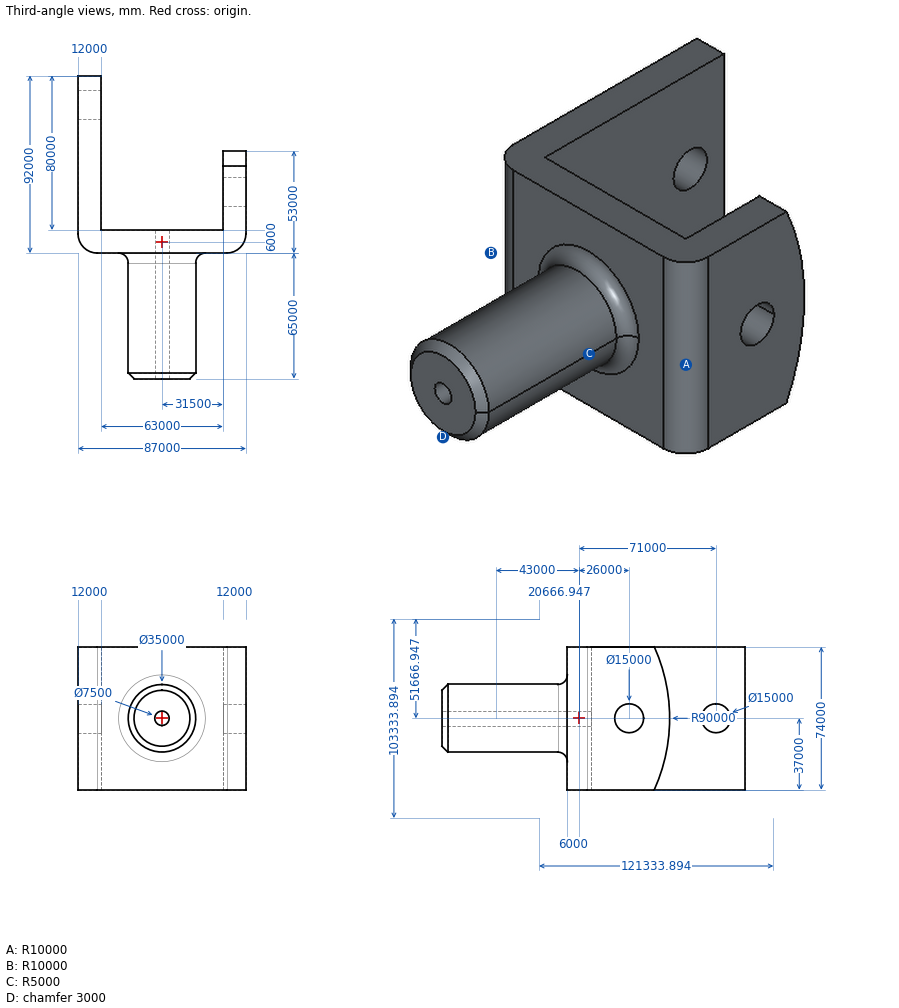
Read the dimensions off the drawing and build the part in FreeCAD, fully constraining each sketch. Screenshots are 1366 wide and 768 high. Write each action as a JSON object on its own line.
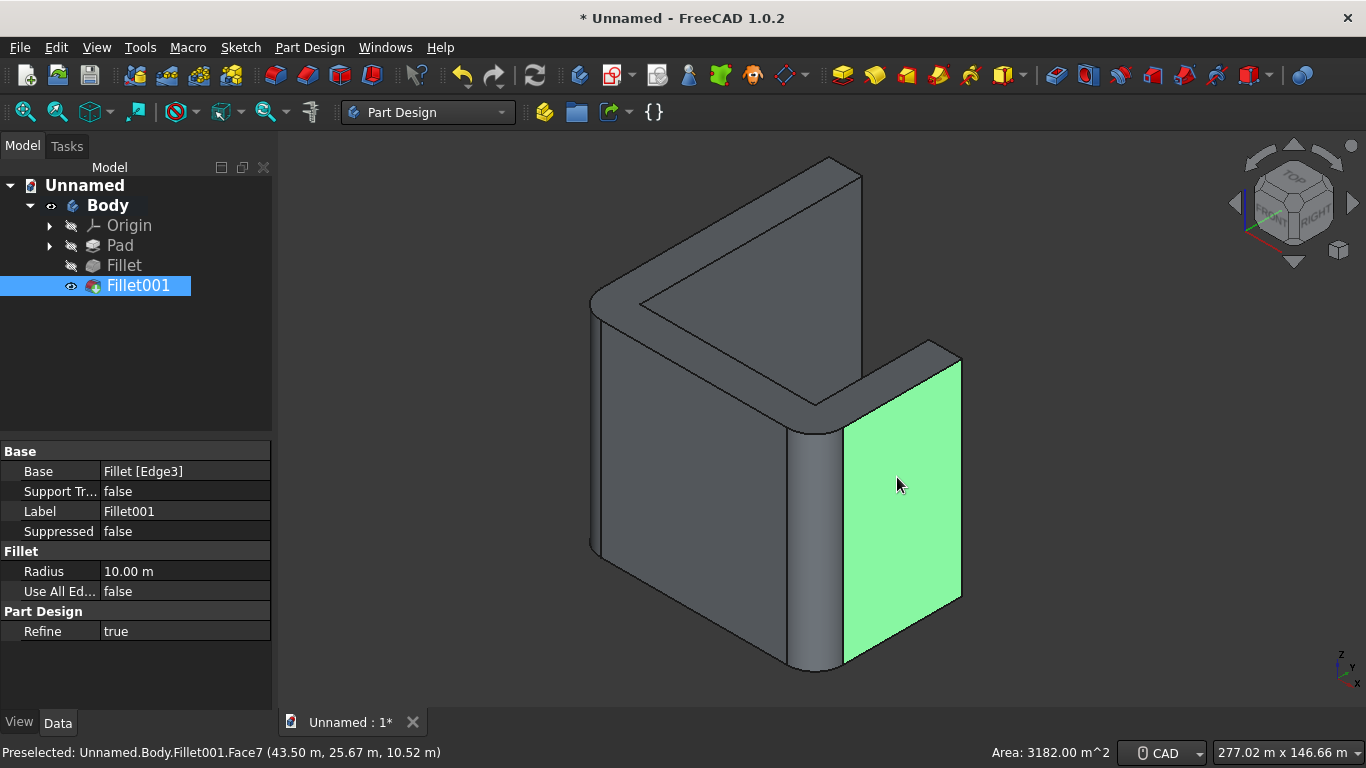
{"action": "left_click", "coordinate": [612, 76]}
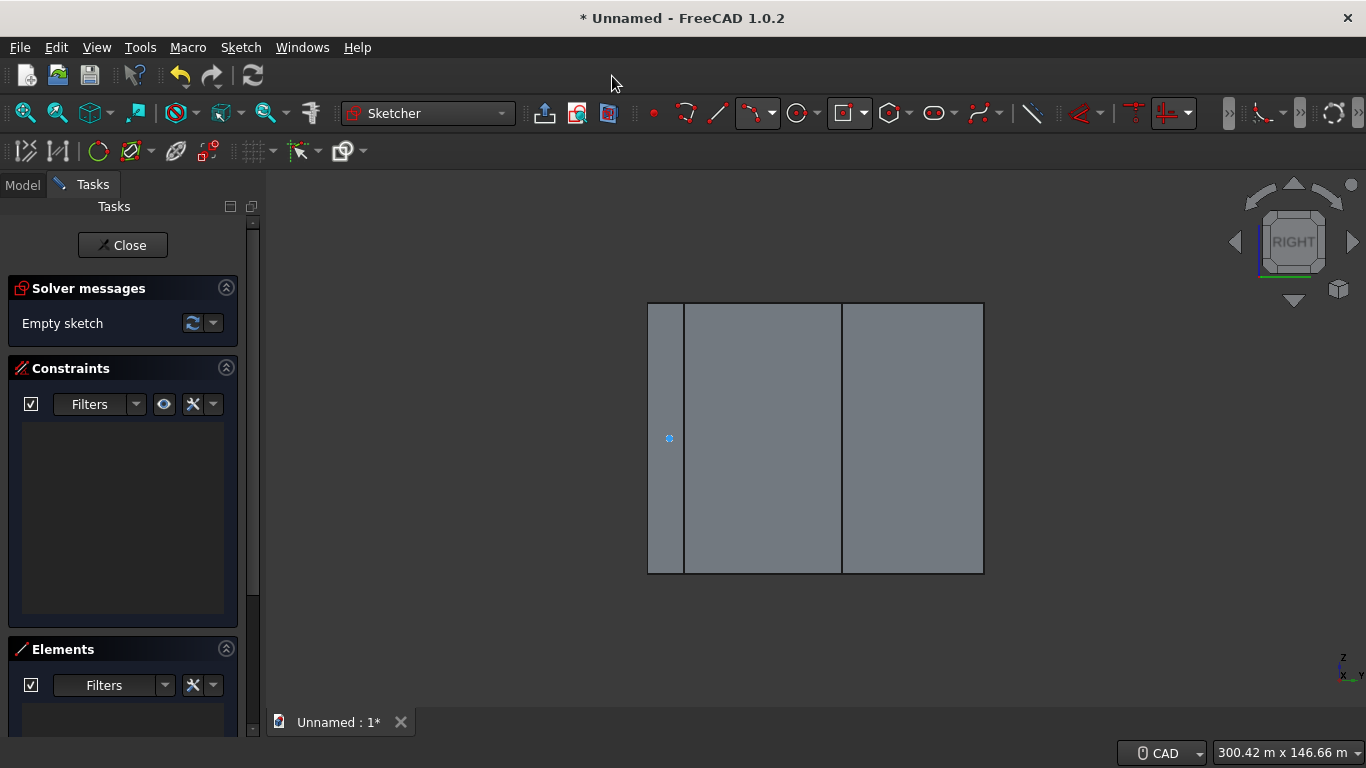
{"action": "key", "text": "g r"}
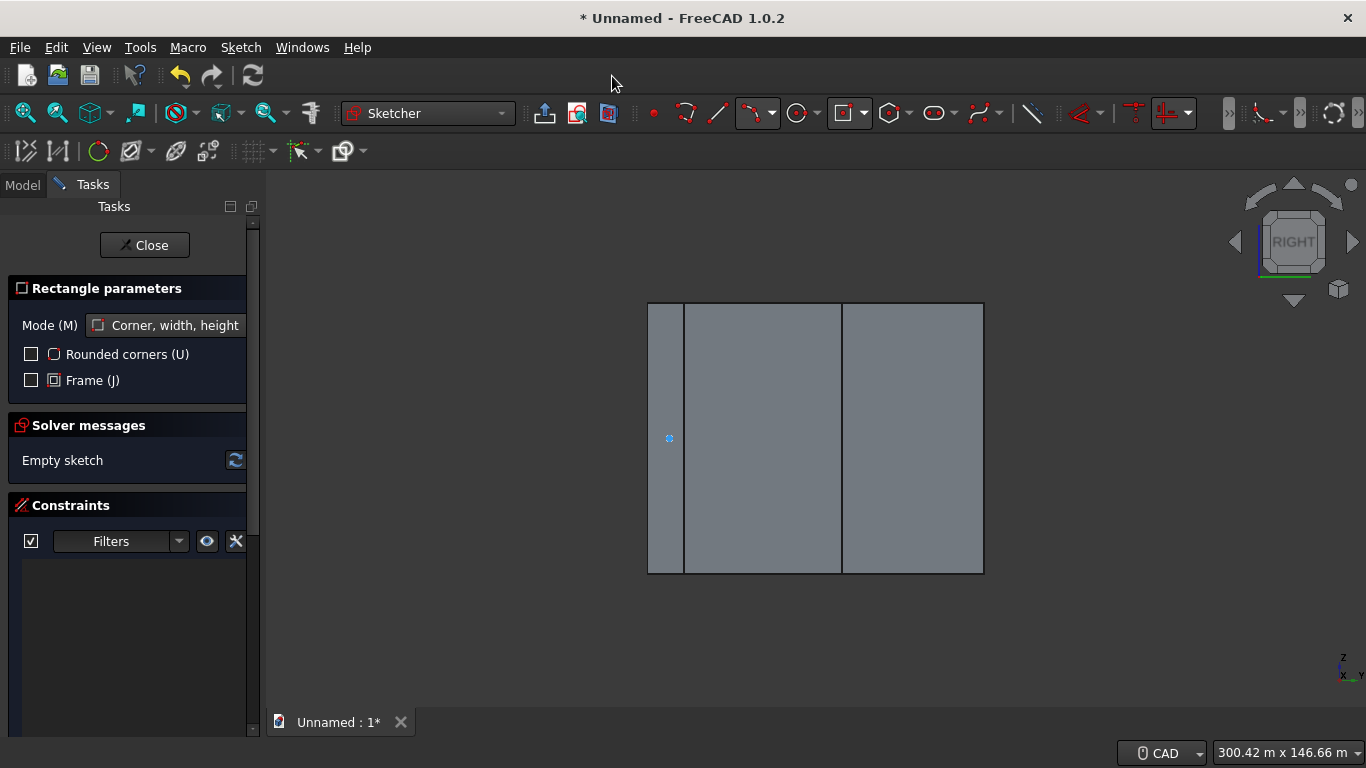
{"action": "left_click", "coordinate": [594, 249]}
{"action": "left_click", "coordinate": [1038, 628]}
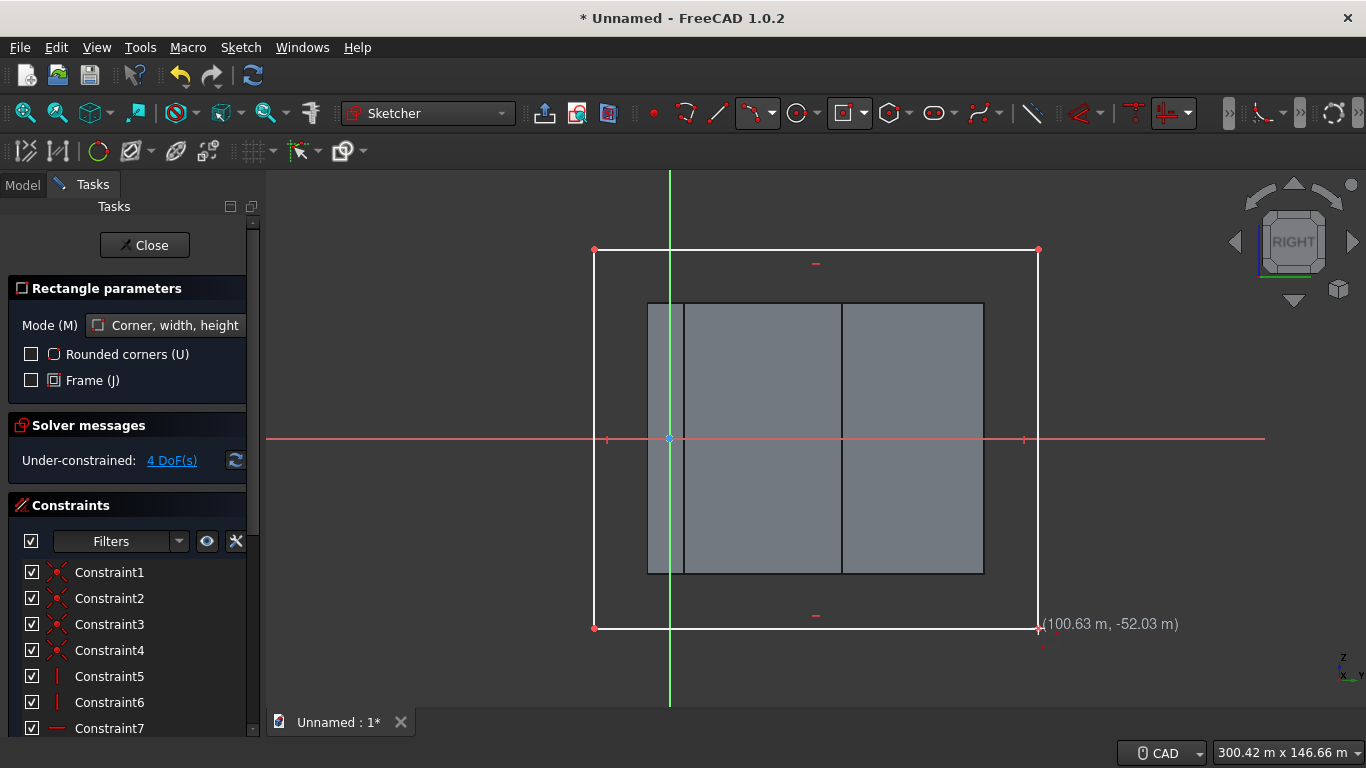
{"action": "left_click", "coordinate": [686, 114]}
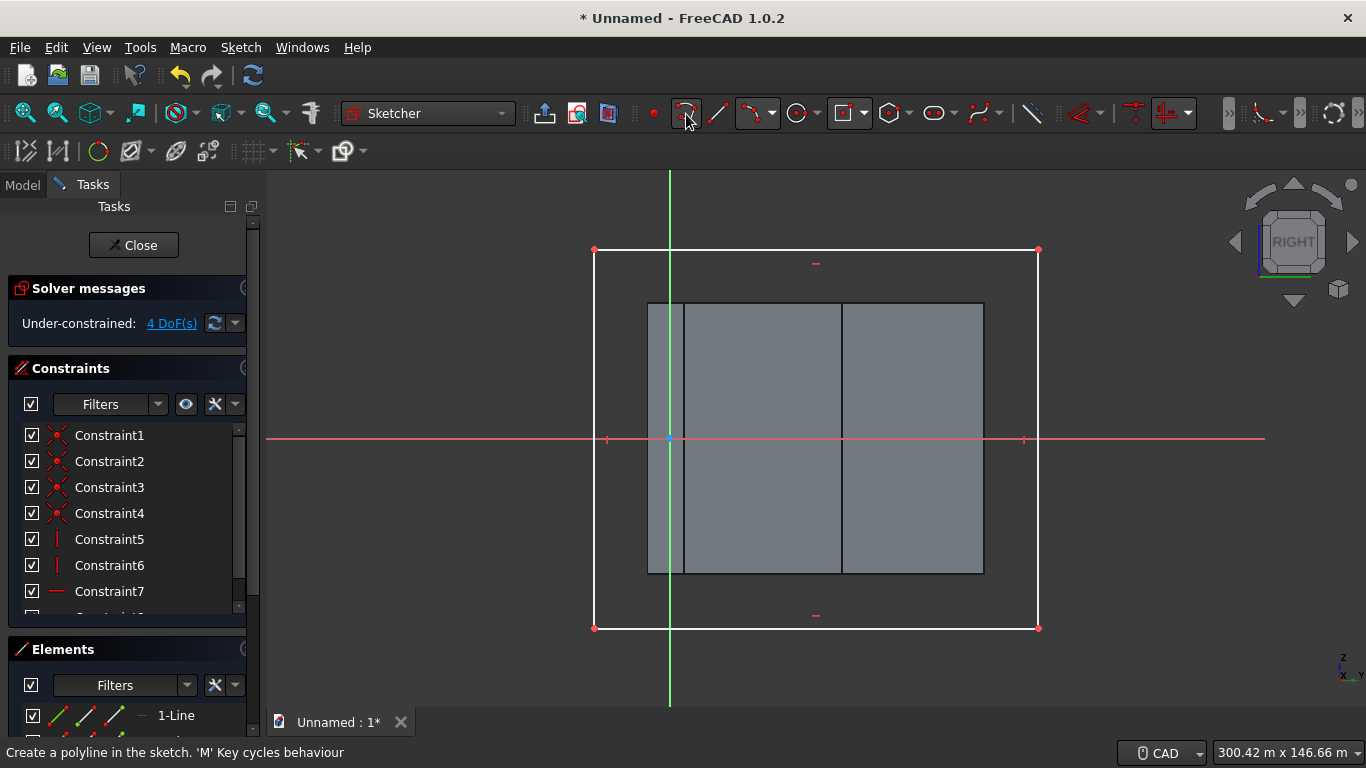
{"action": "left_click", "coordinate": [812, 574]}
{"action": "left_click", "coordinate": [648, 574]}
{"action": "left_click", "coordinate": [648, 303]}
{"action": "left_click", "coordinate": [812, 303]}
{"action": "right_click", "coordinate": [812, 303]}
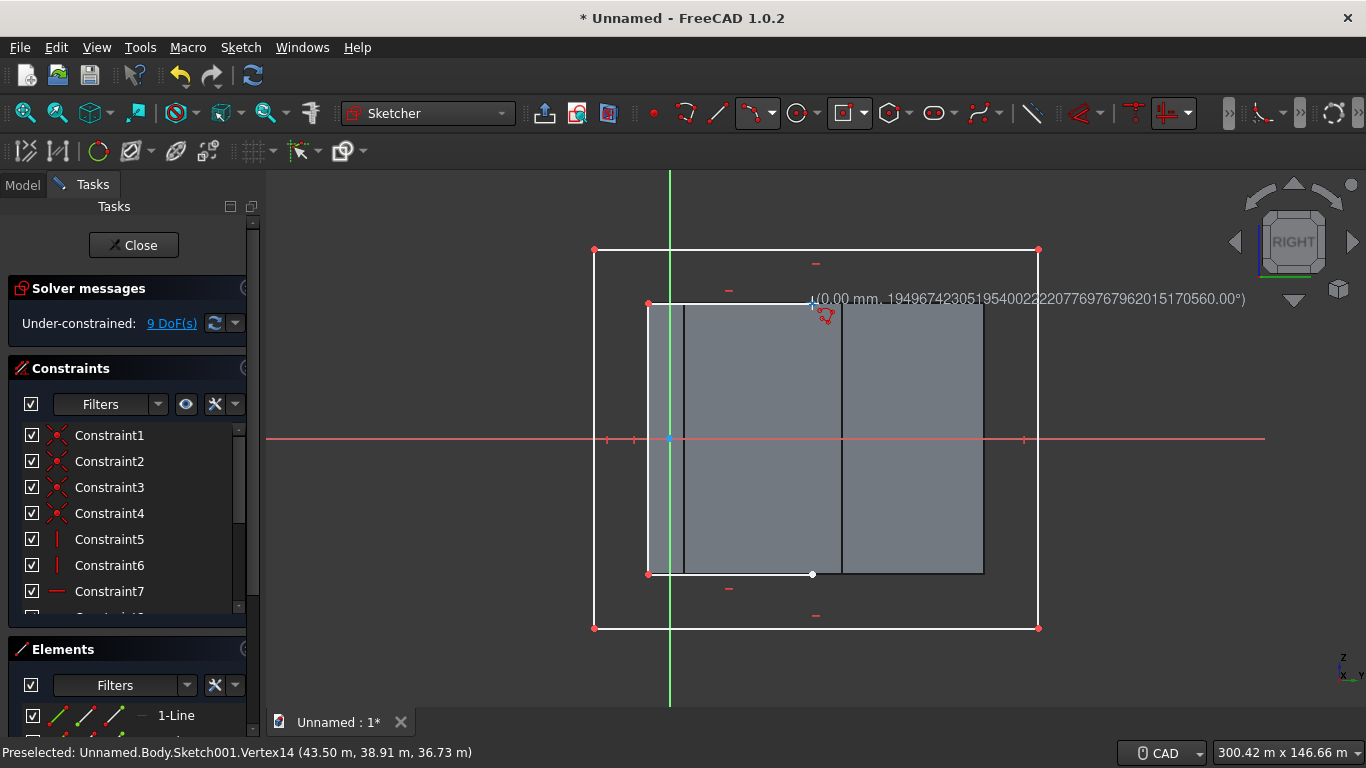
{"action": "left_click", "coordinate": [752, 114]}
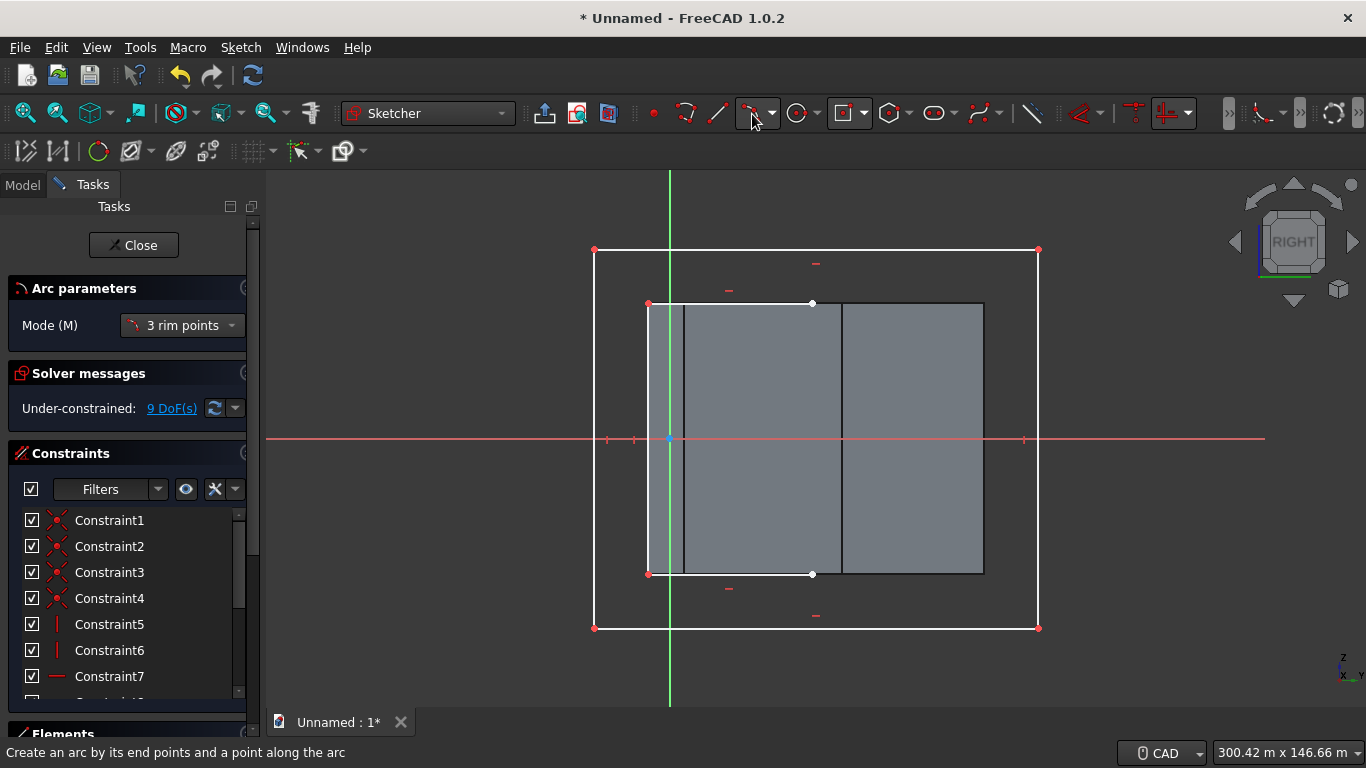
{"action": "left_click", "coordinate": [812, 304]}
{"action": "left_click", "coordinate": [812, 575]}
{"action": "left_click", "coordinate": [840, 466]}
{"action": "key", "text": "Escape"}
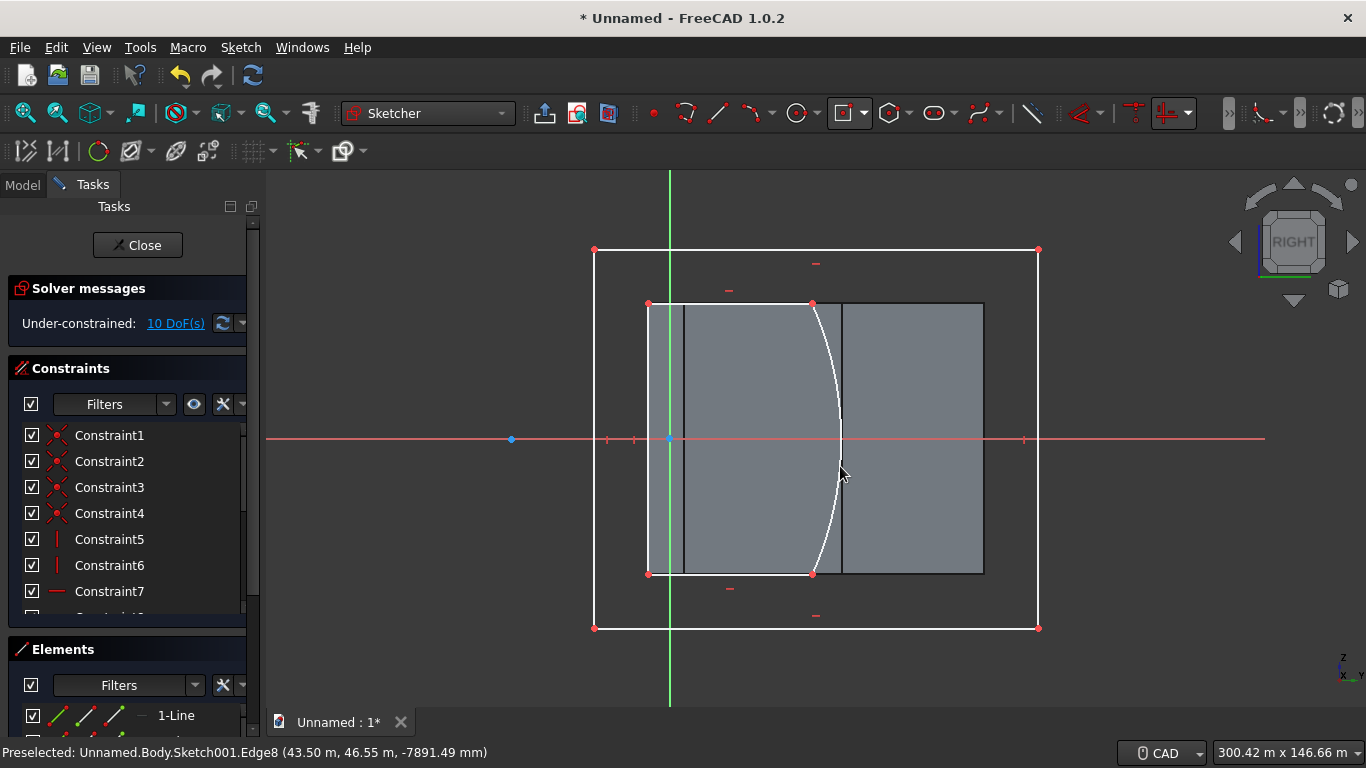
{"action": "left_click", "coordinate": [512, 439]}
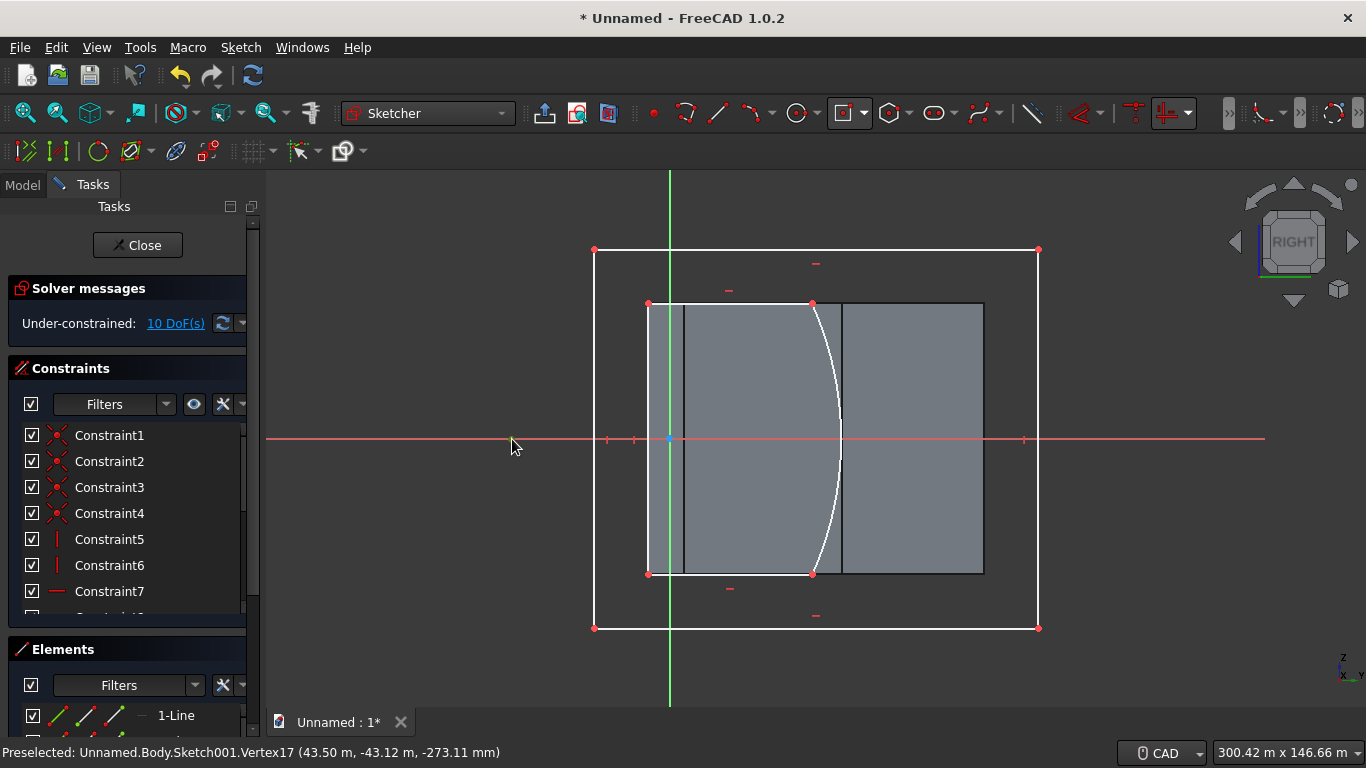
{"action": "left_click", "coordinate": [359, 438]}